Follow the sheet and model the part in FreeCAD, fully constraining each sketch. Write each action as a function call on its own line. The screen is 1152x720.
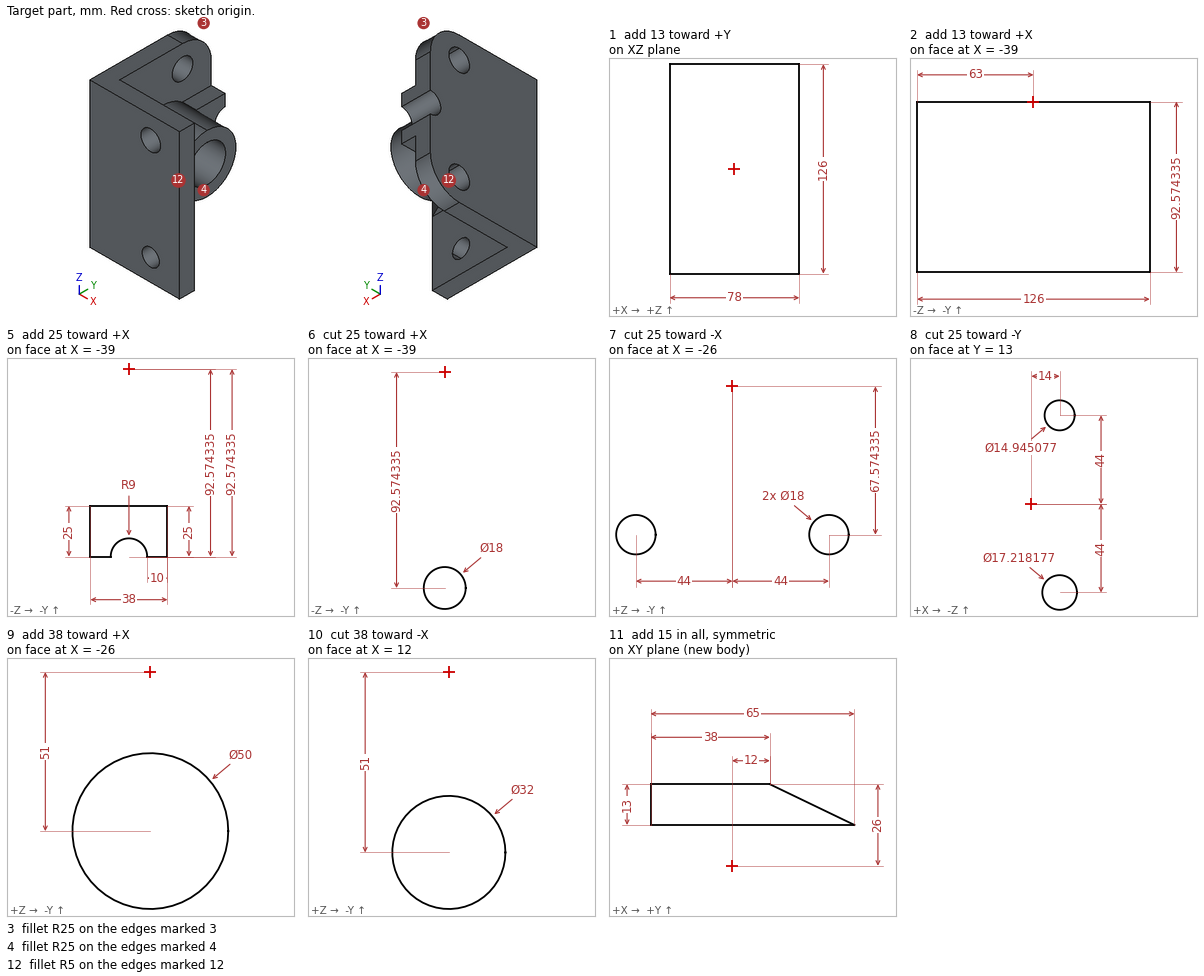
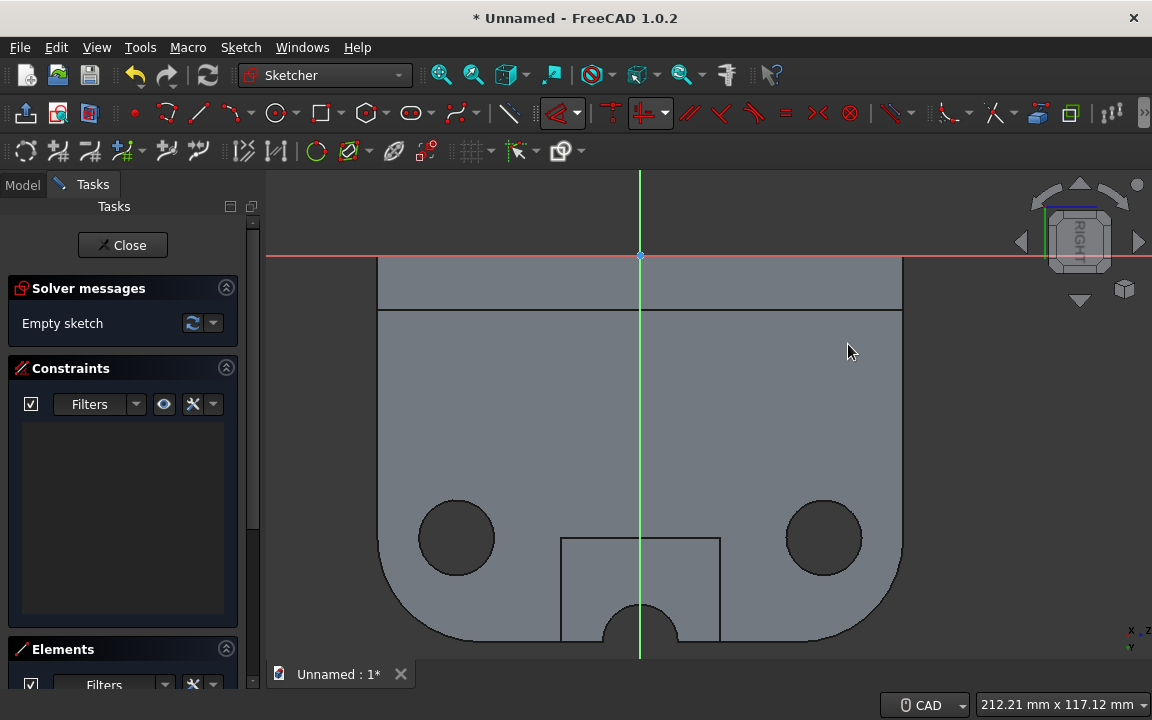
key(g)
key(c)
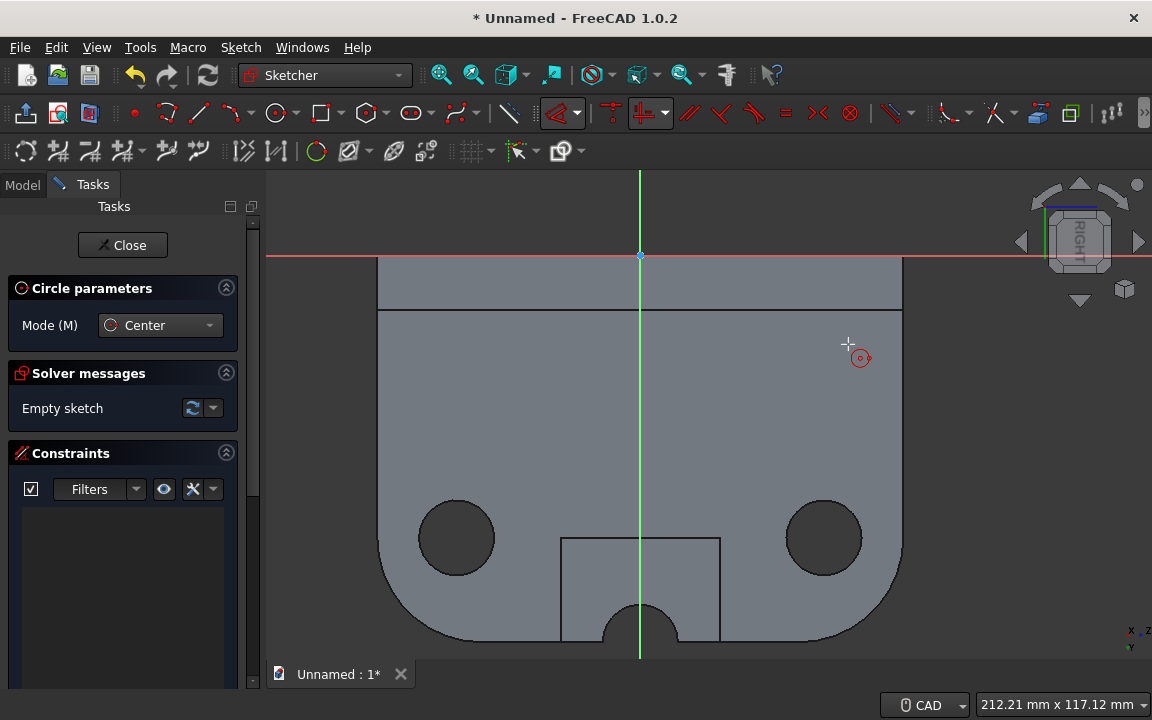
click(640, 469)
move(714, 395)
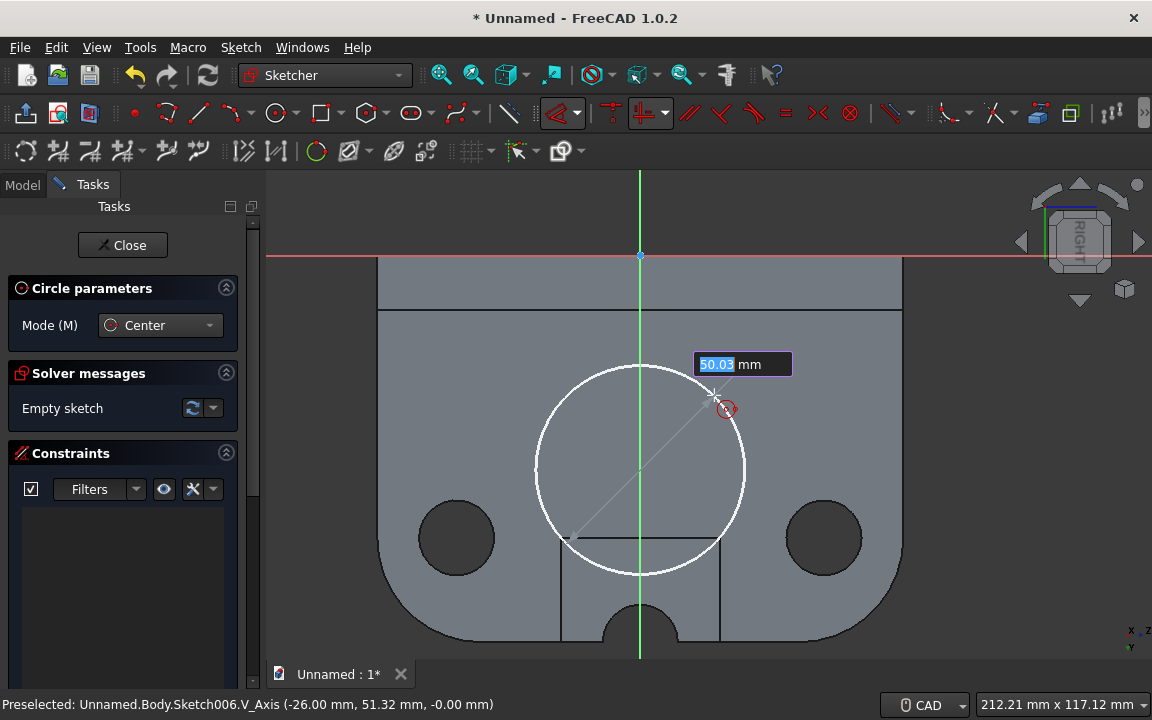
text(50)
key(Return)
key(Escape)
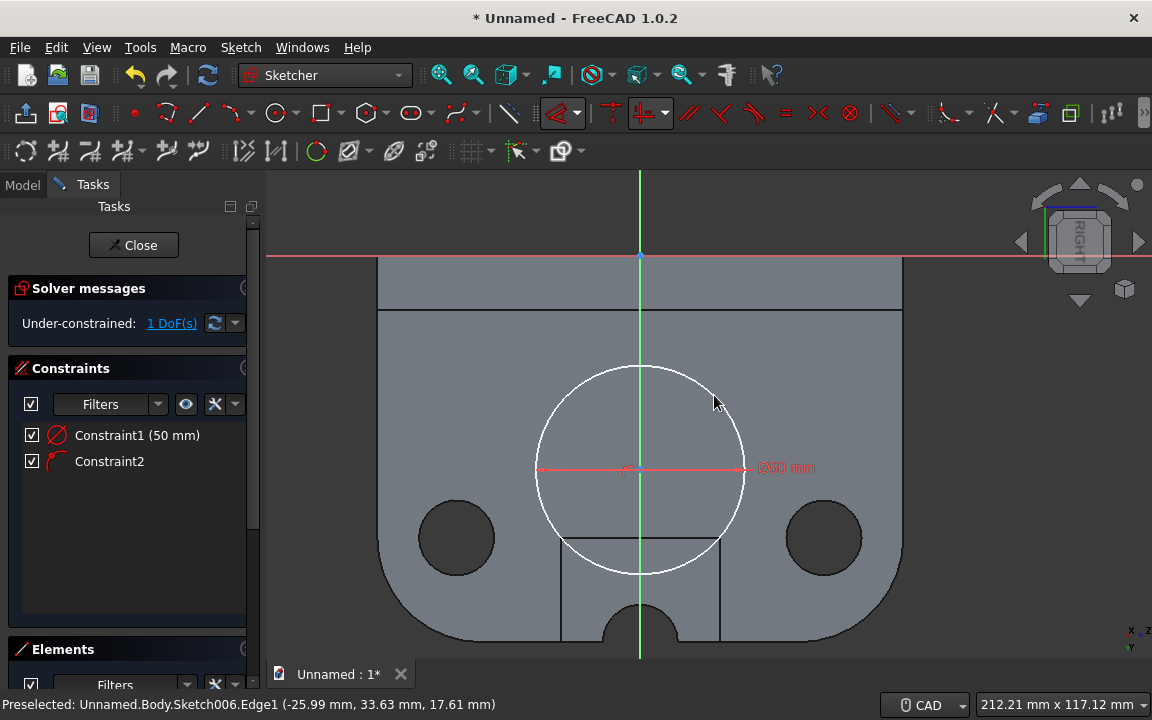
click(640, 470)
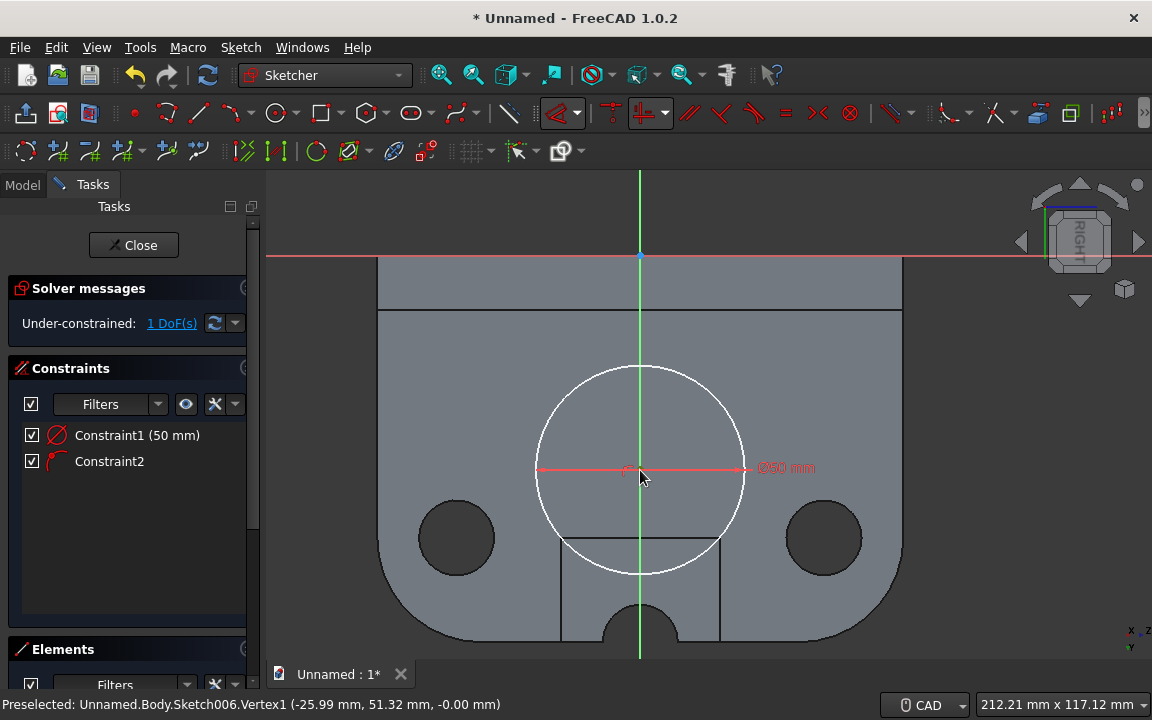
key(i)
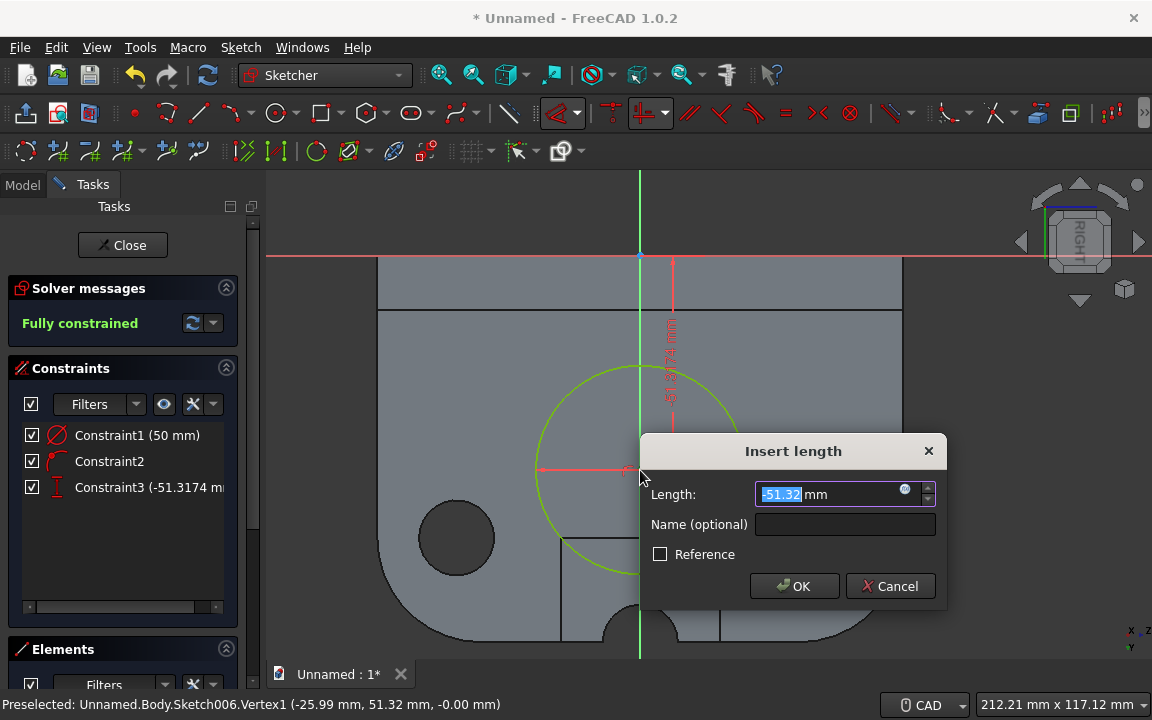
text(-51)
key(Return)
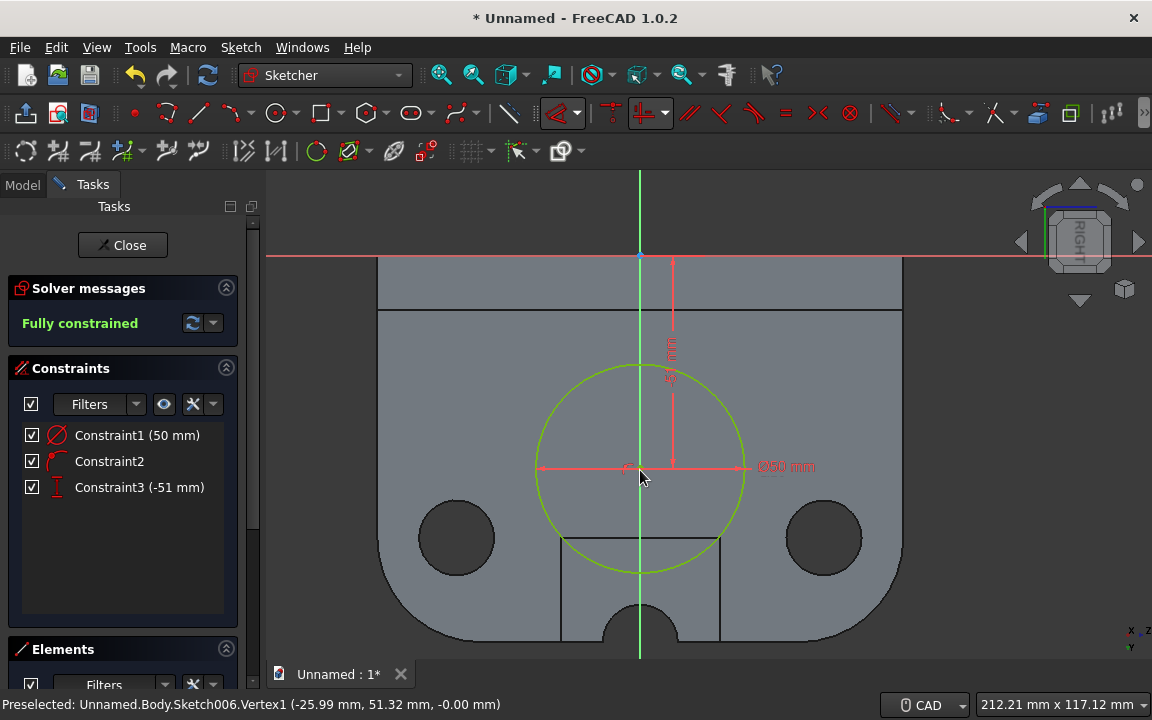
click(123, 245)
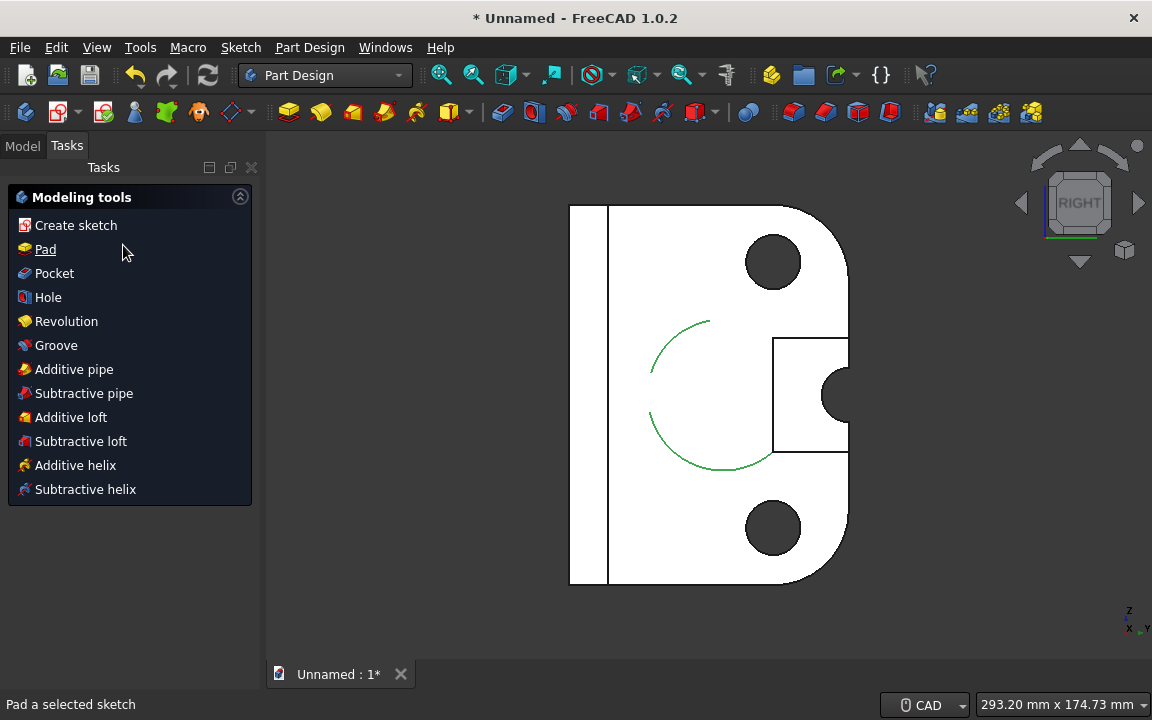
click(290, 112)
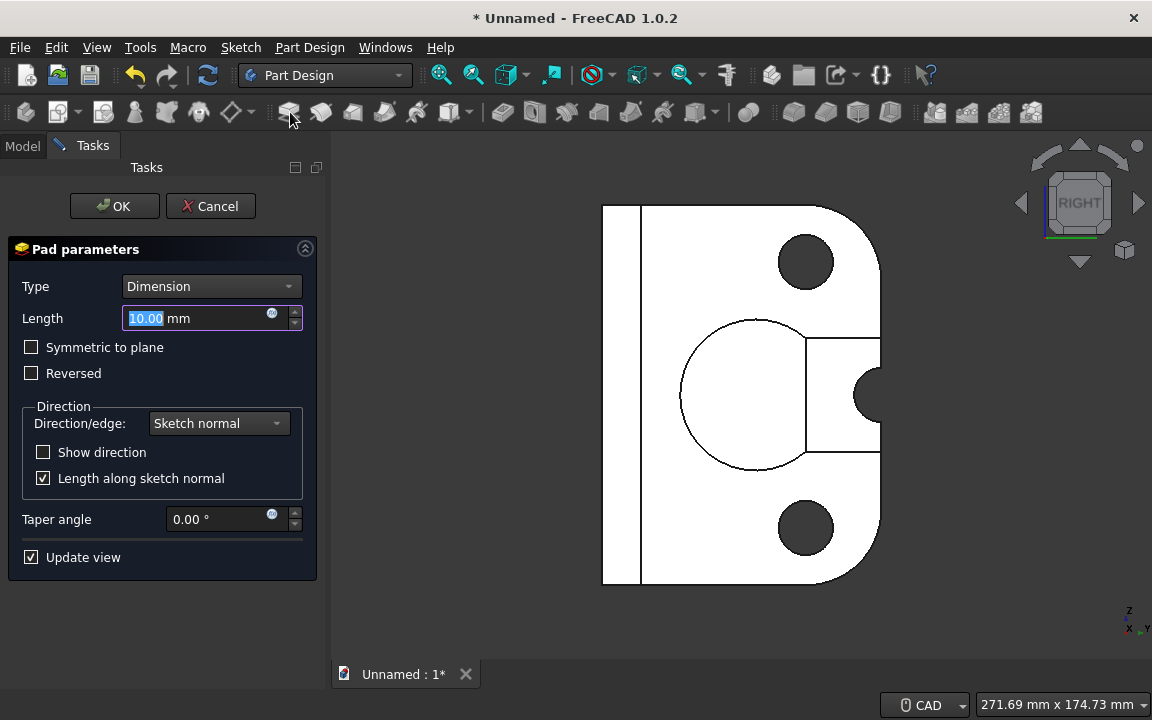
text(38)
key(Tab)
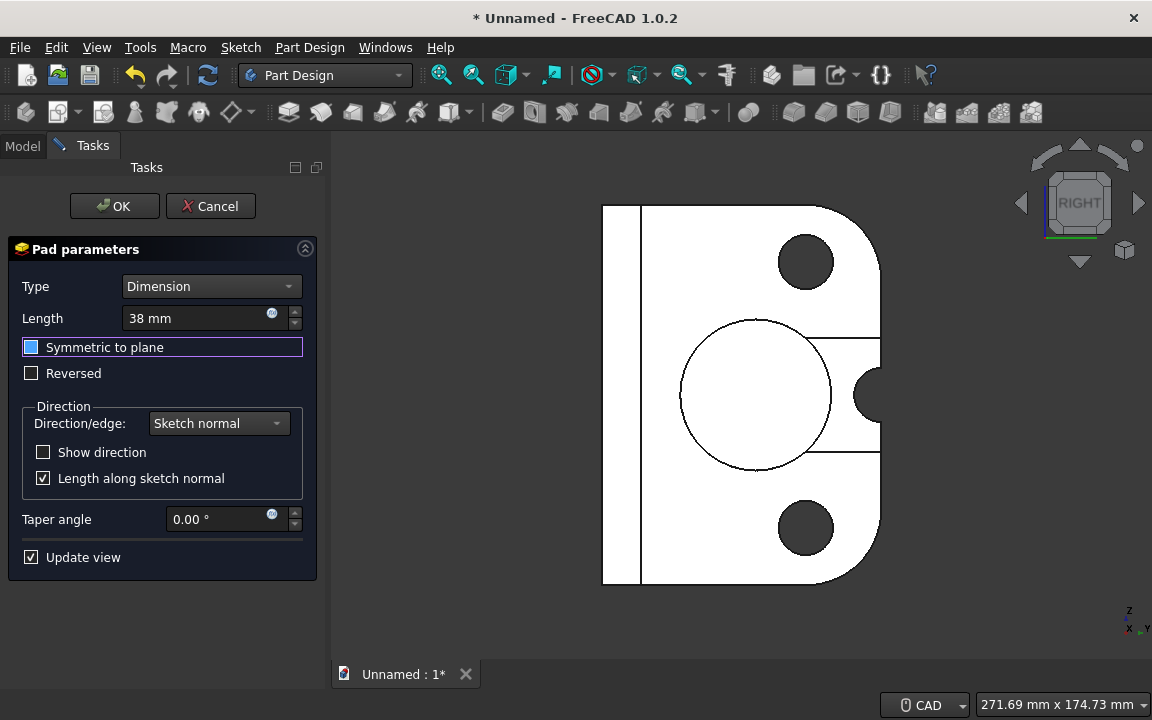
click(115, 206)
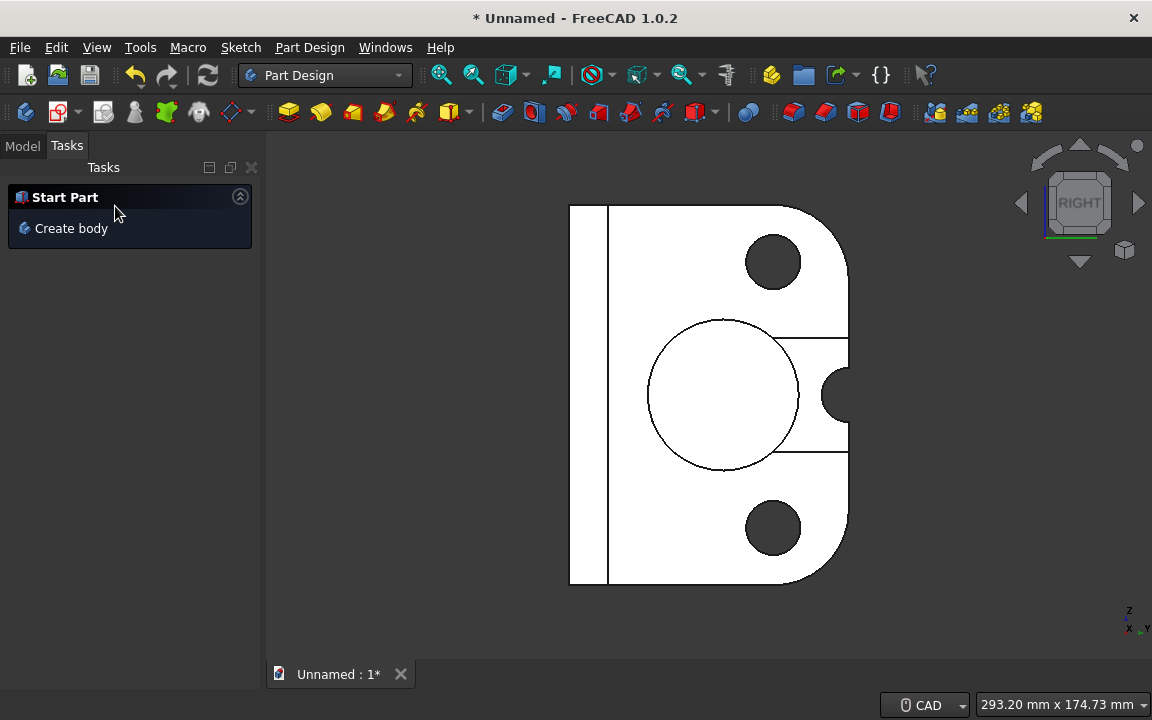
click(723, 394)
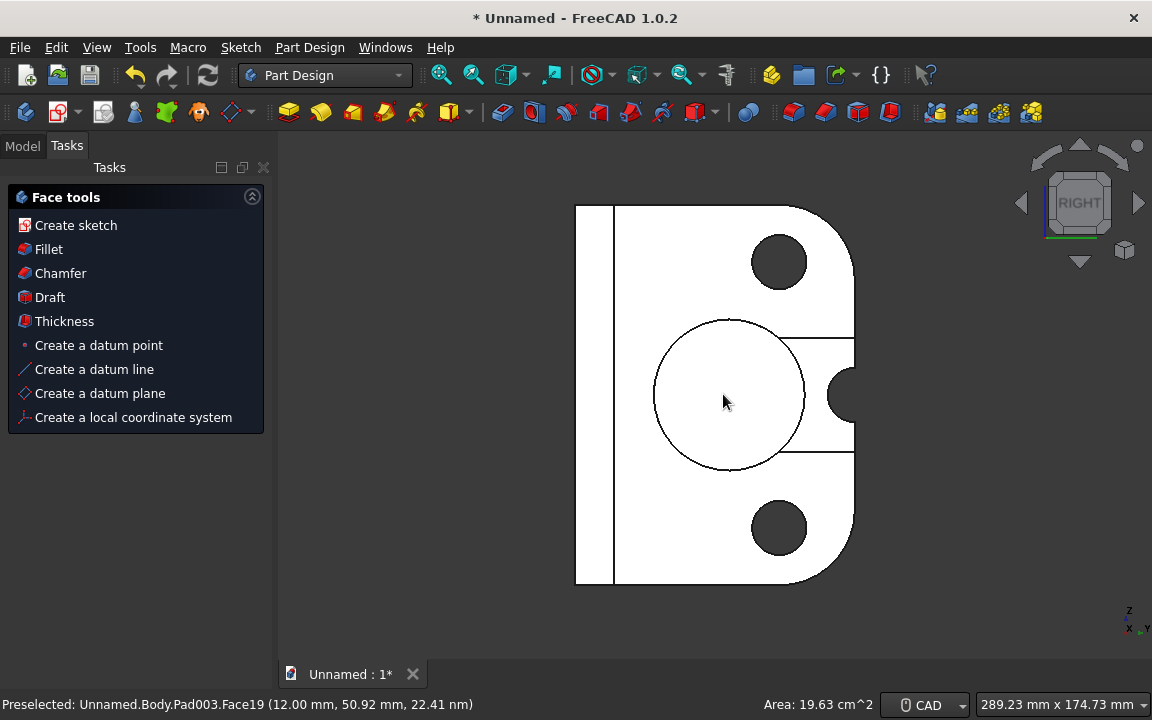
click(58, 112)